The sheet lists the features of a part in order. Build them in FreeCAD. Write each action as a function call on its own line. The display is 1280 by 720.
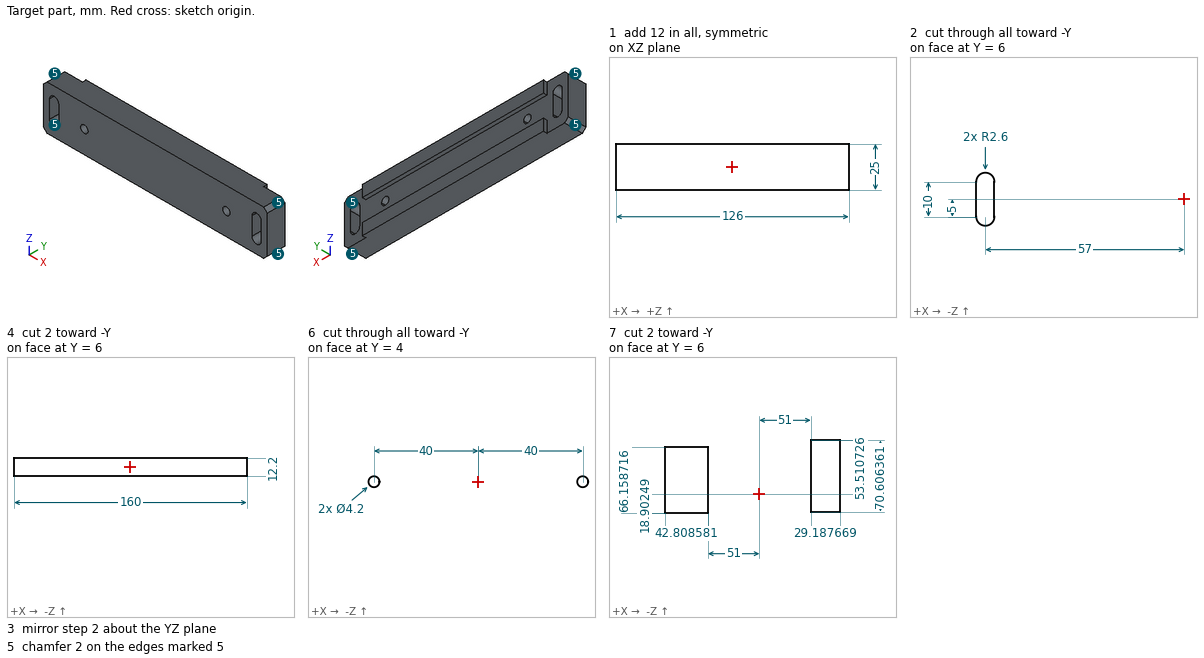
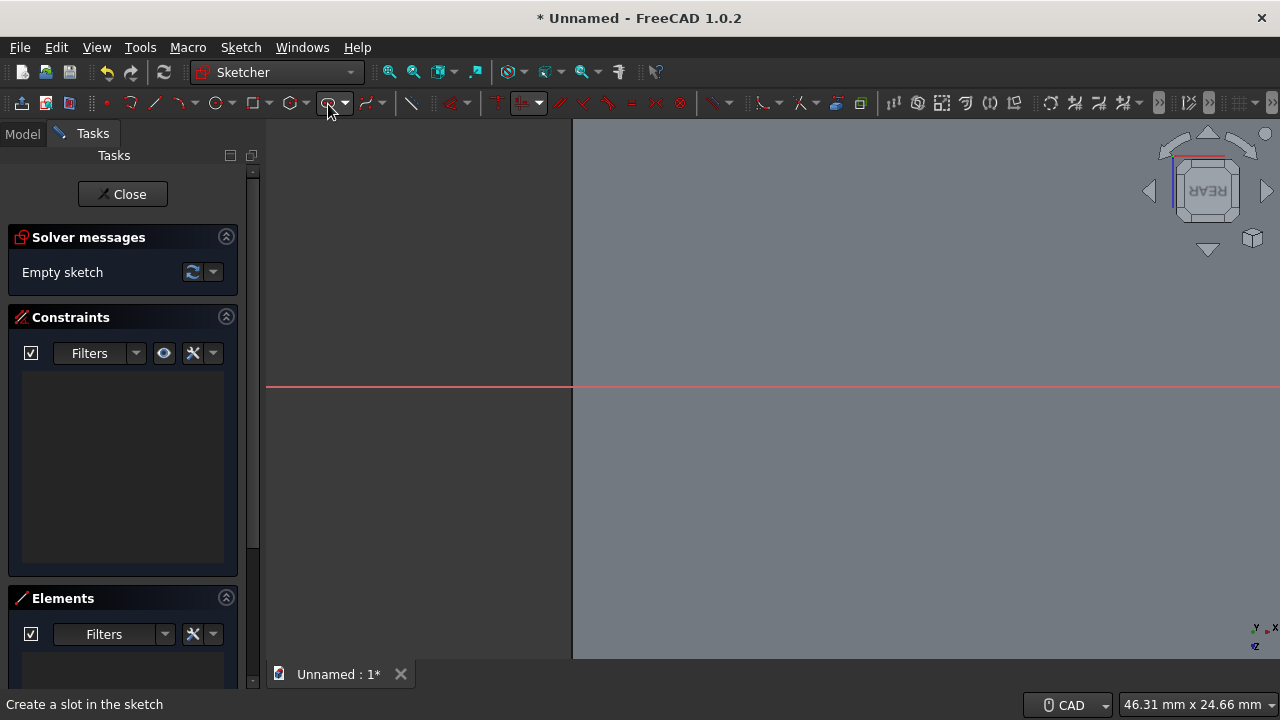
click(704, 497)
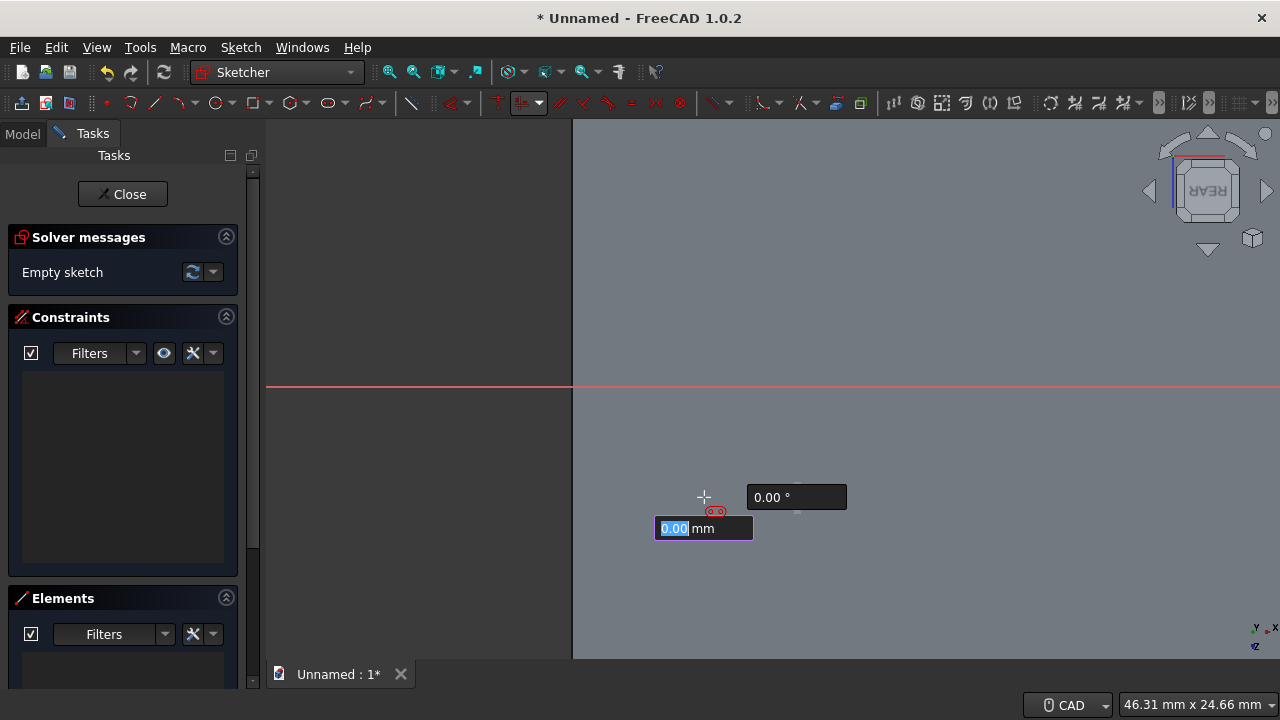
click(704, 278)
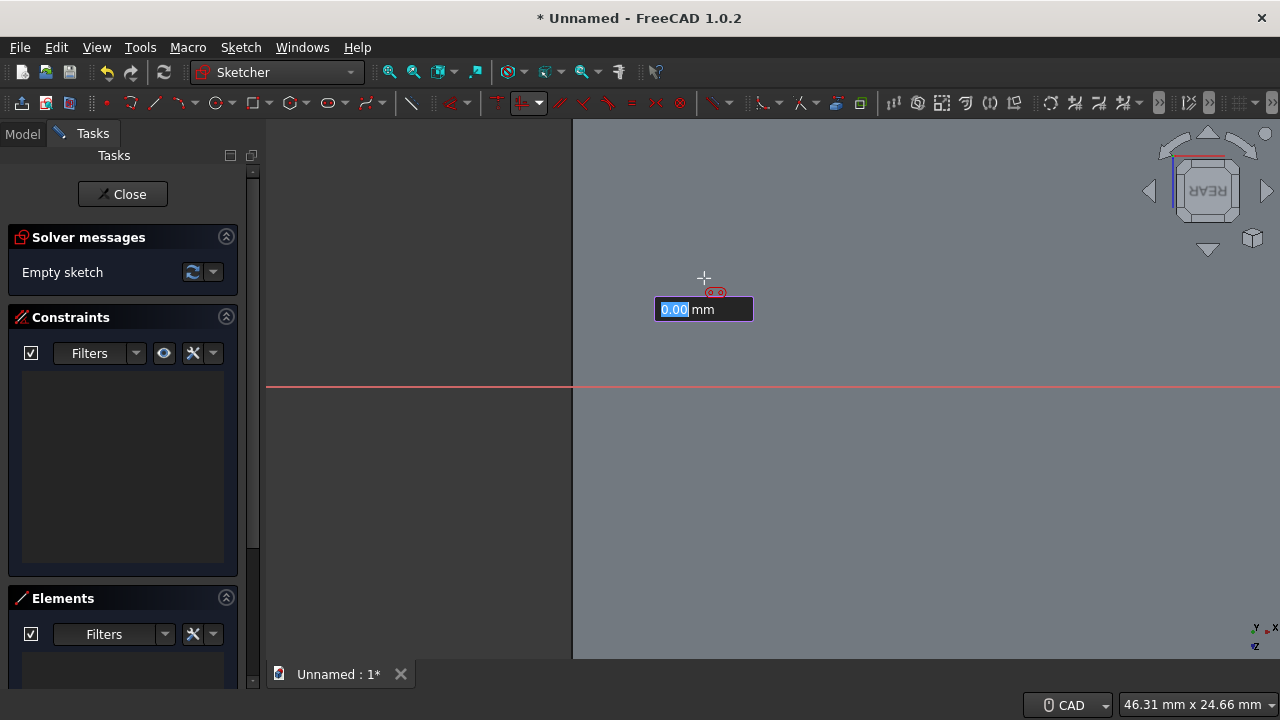
click(761, 420)
key(Escape)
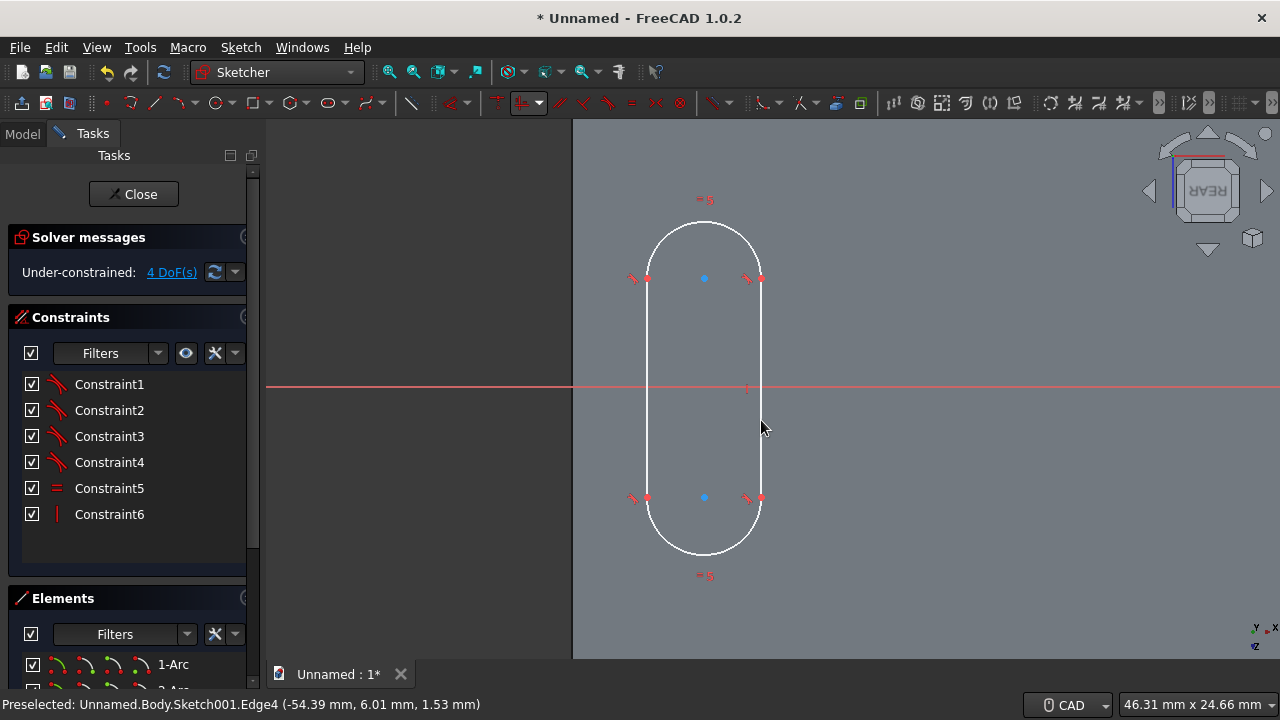
click(450, 104)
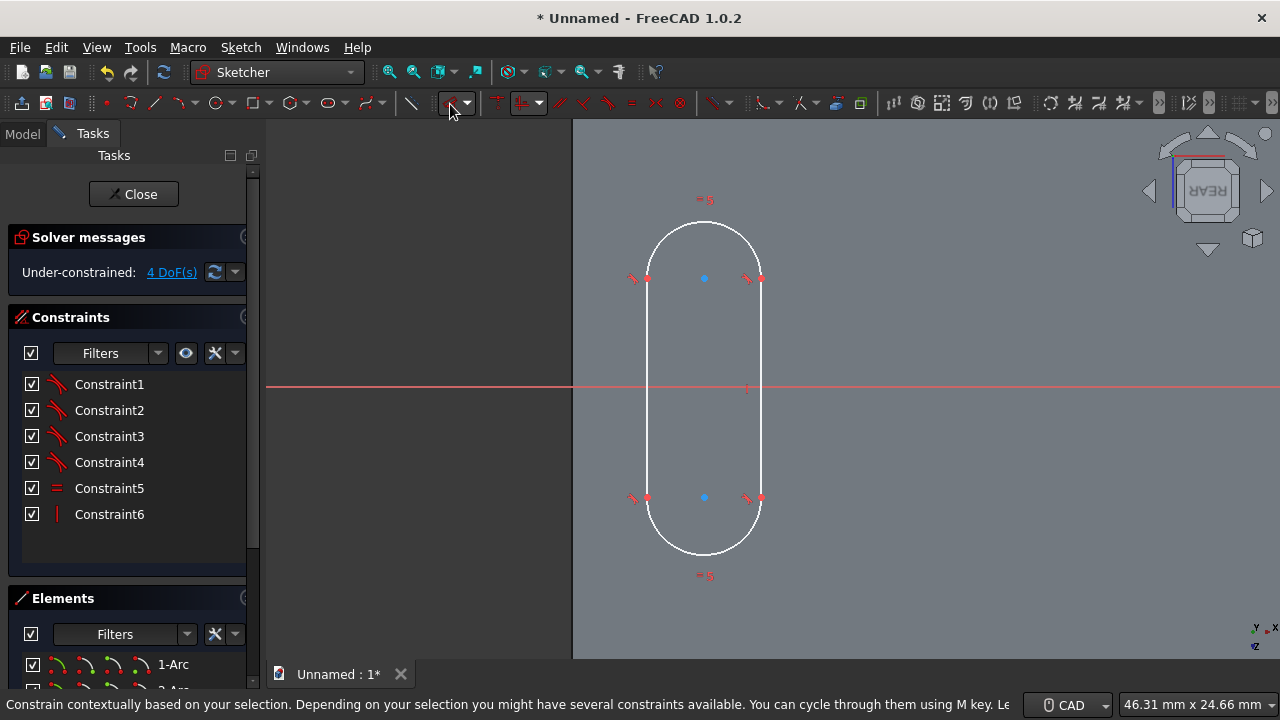
click(670, 544)
click(651, 570)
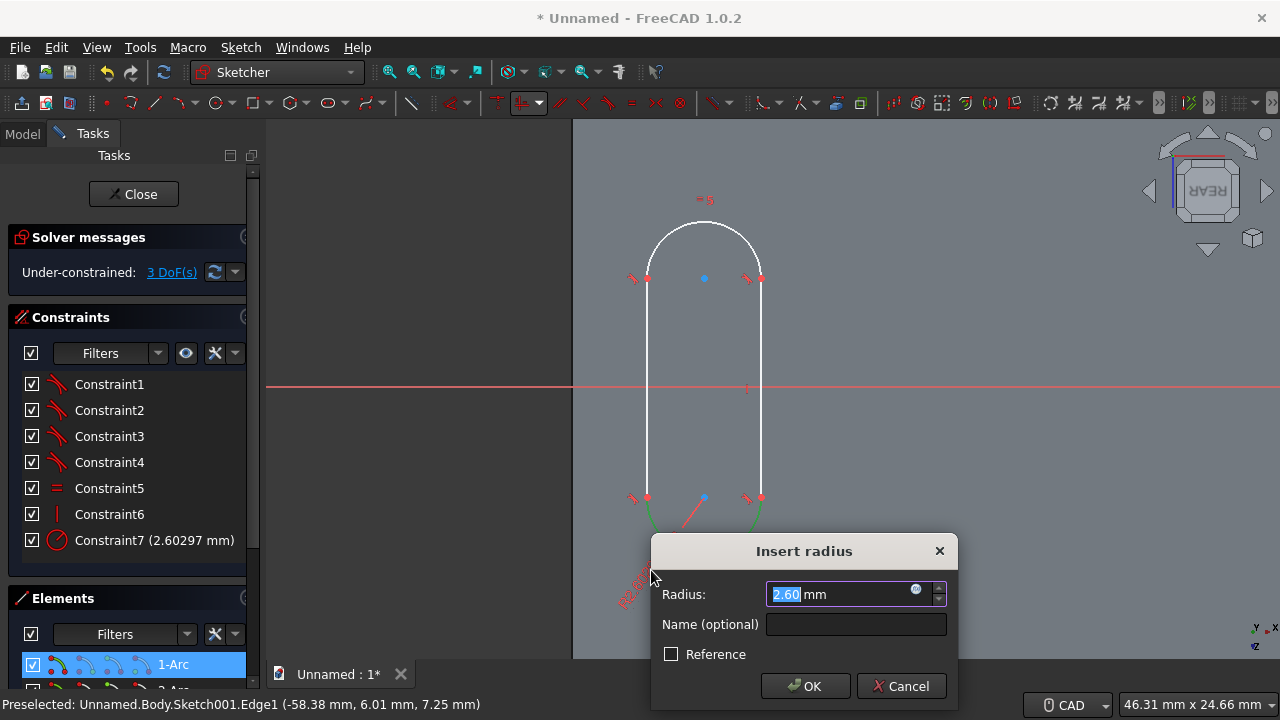
text(2.6)
key(Return)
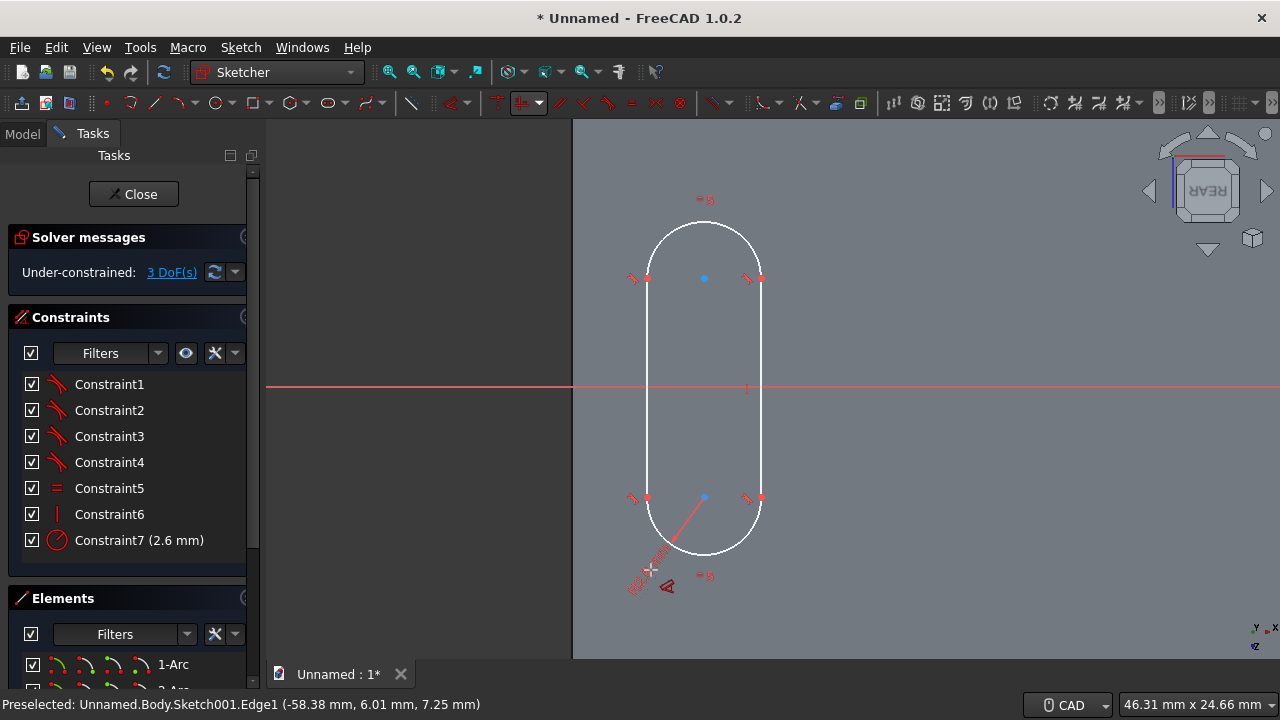
click(647, 432)
click(613, 338)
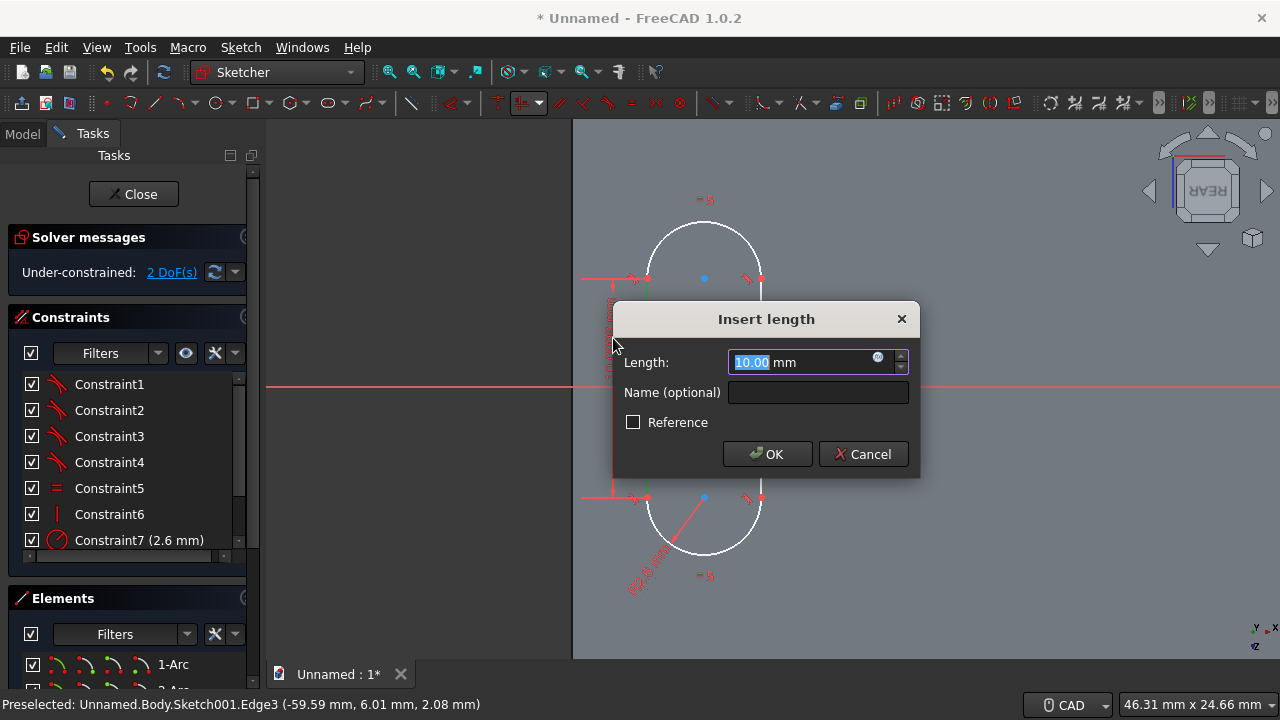
text(10)
key(Return)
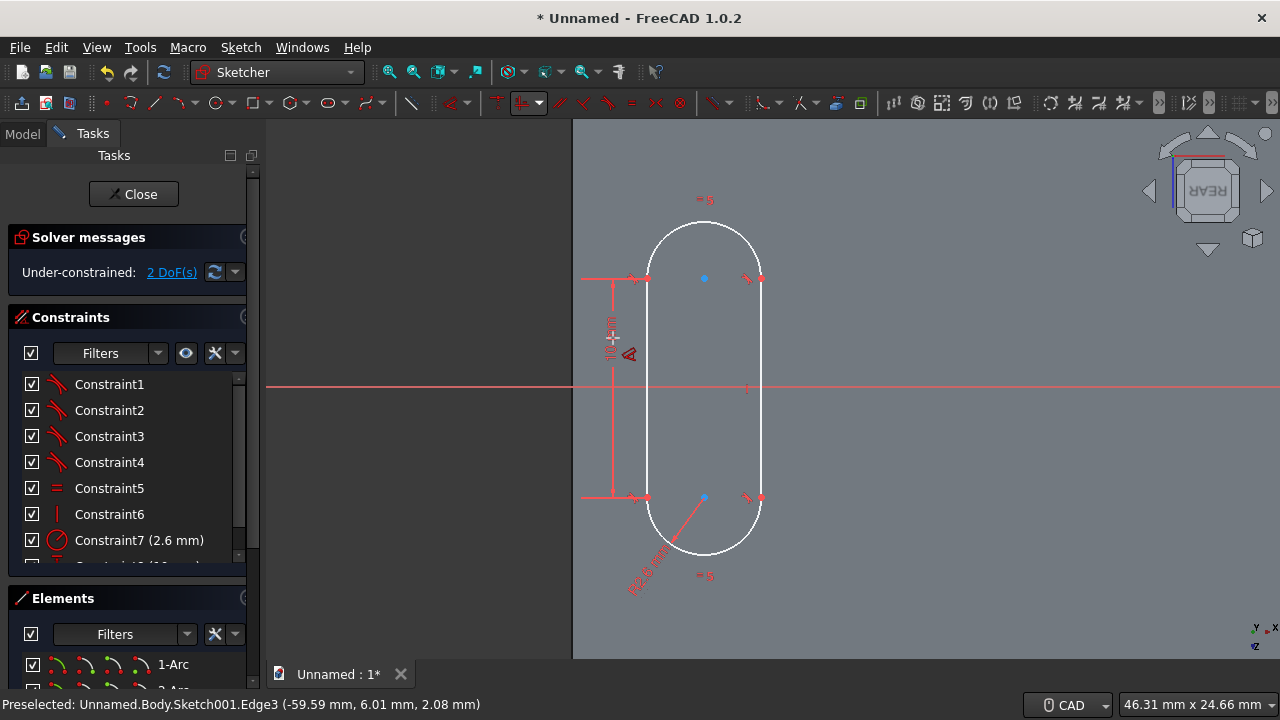
click(647, 498)
click(613, 443)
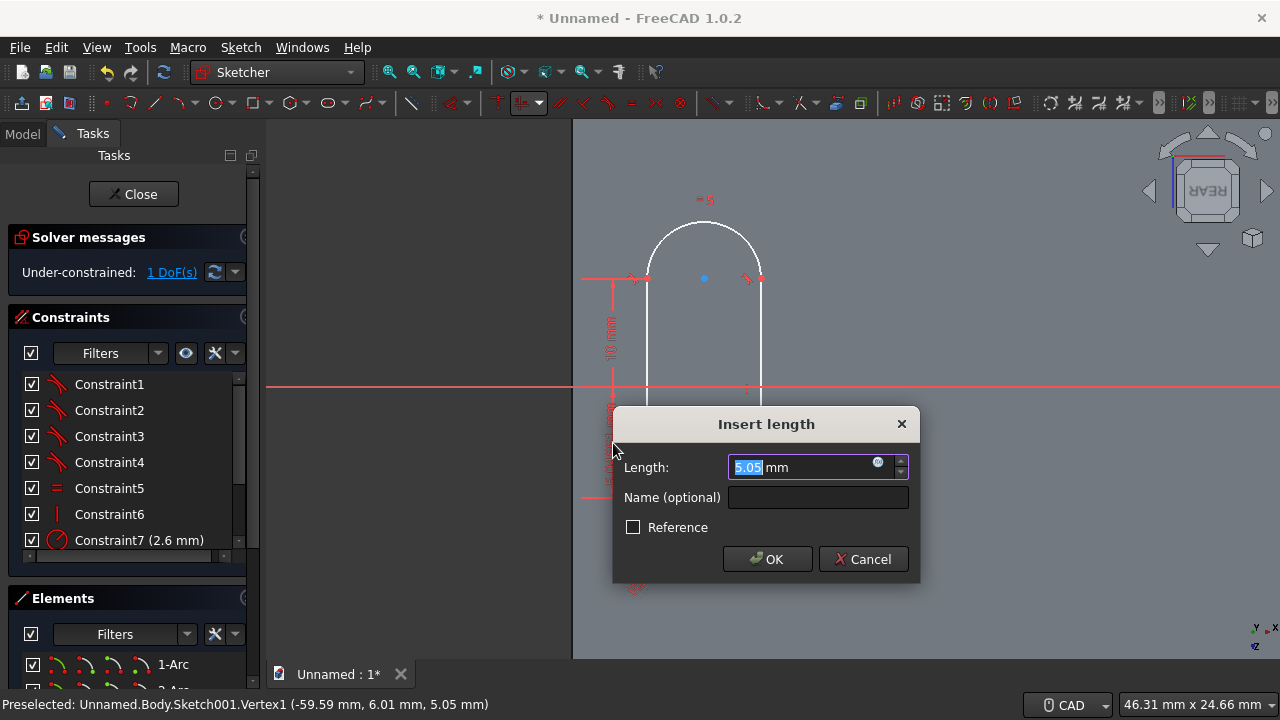
text(5)
key(Return)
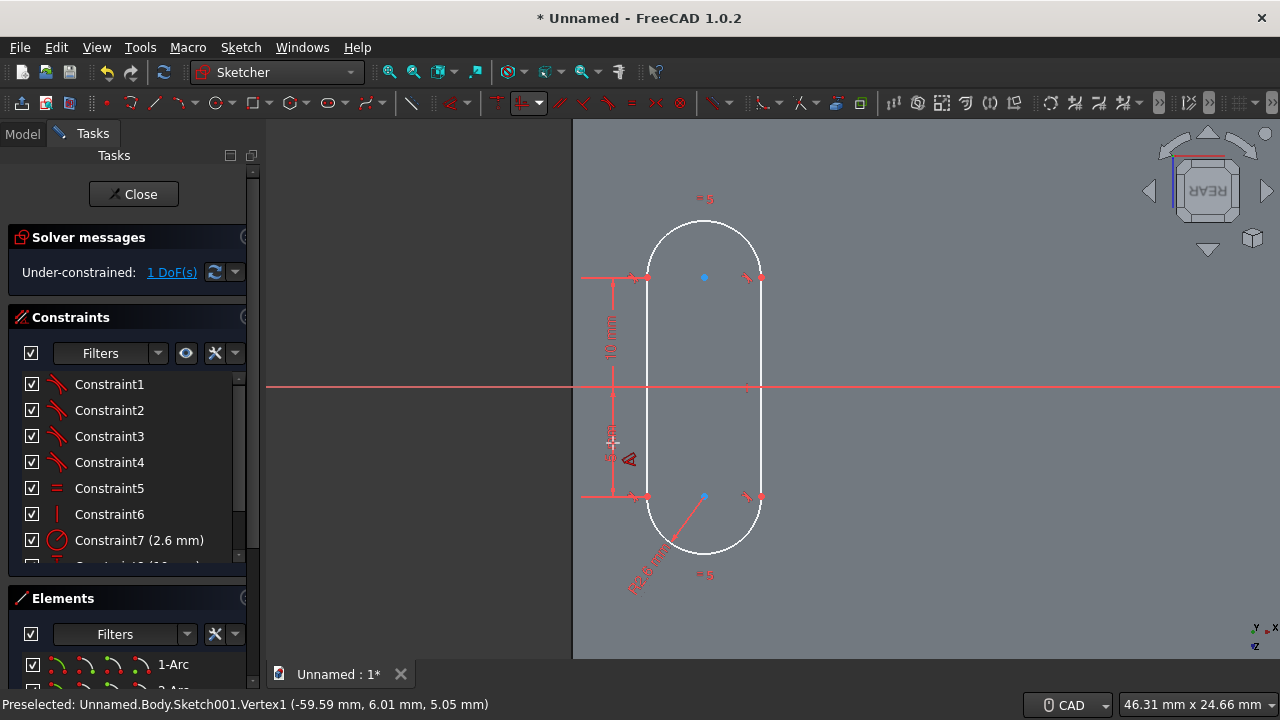
click(704, 497)
click(910, 531)